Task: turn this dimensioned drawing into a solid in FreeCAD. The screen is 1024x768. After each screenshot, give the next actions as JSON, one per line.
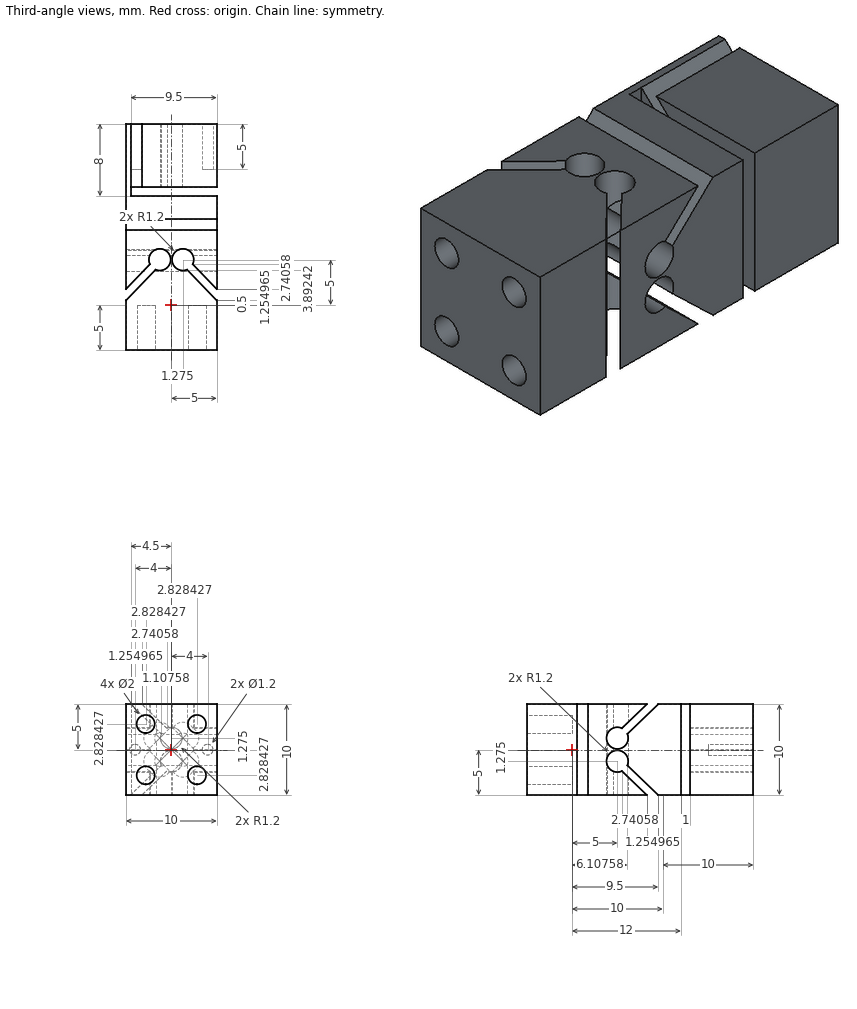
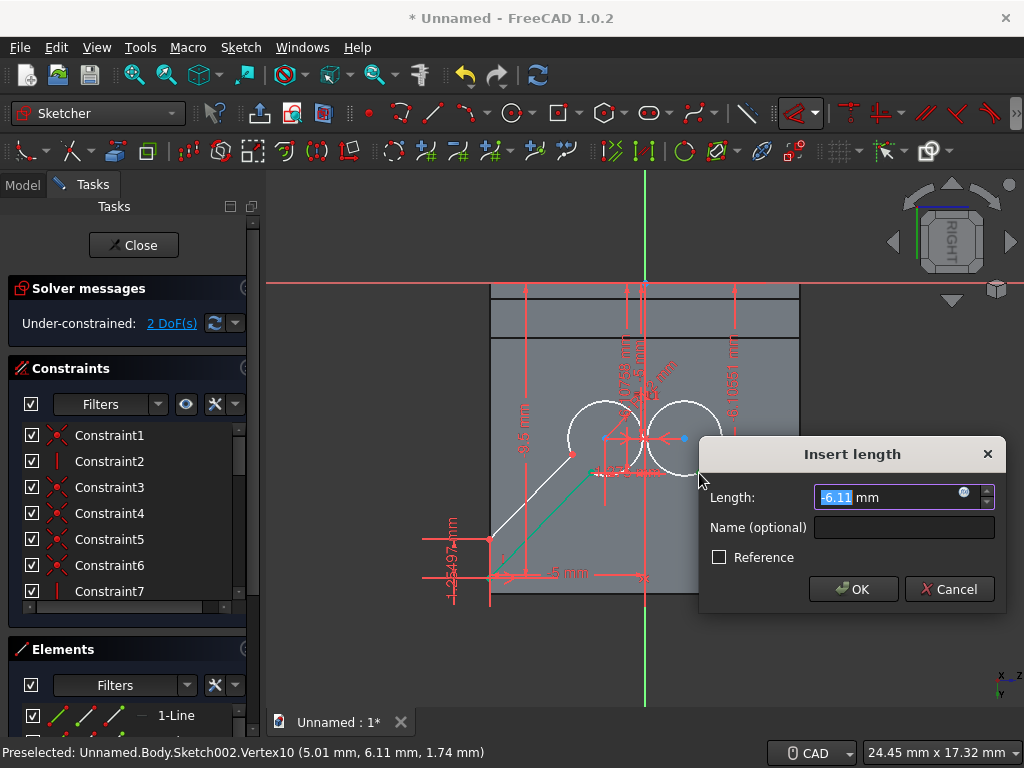
{"action": "type", "text": "-6.10758"}
{"action": "key", "text": "Return"}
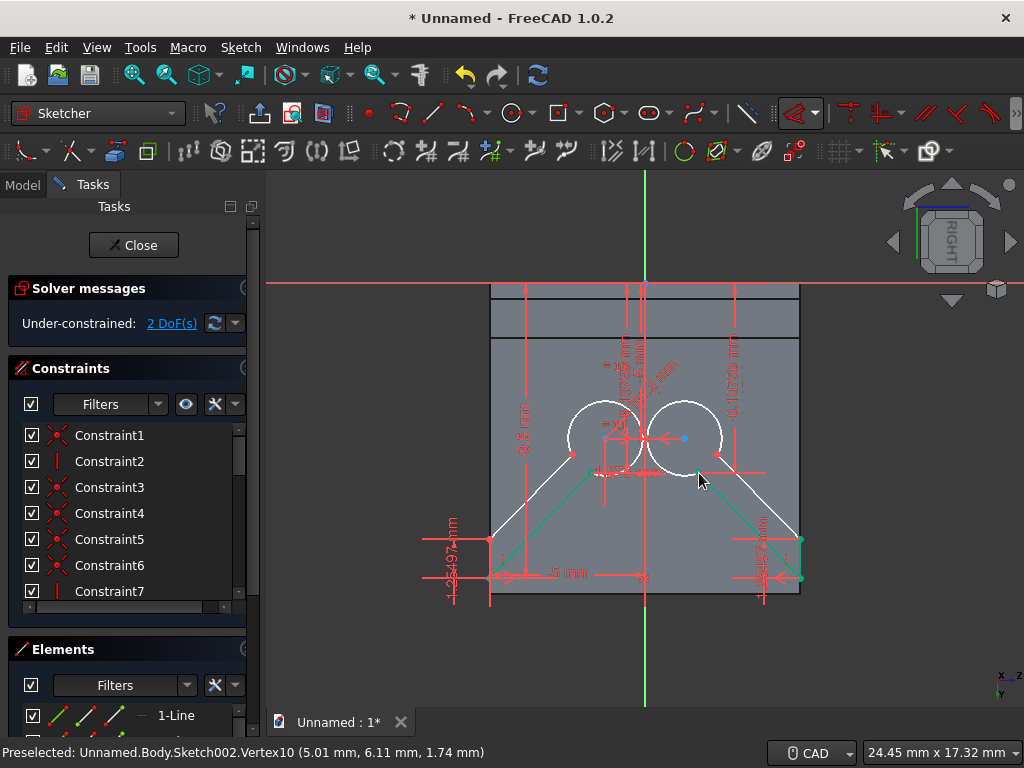
{"action": "left_click", "coordinate": [547, 480]}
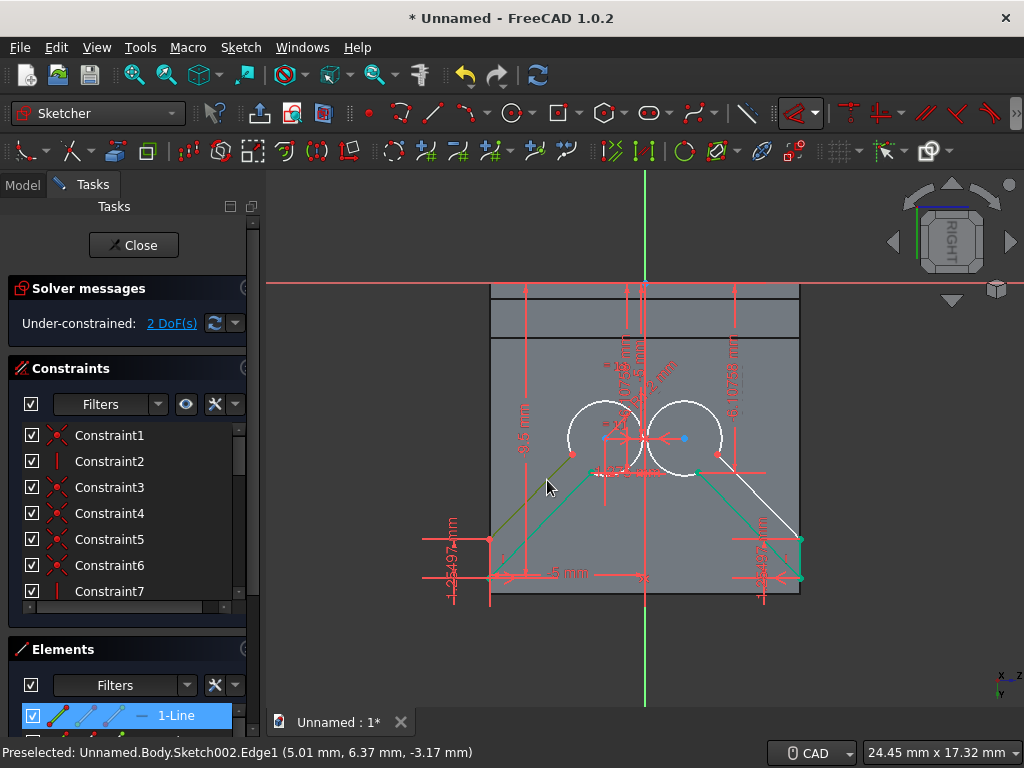
{"action": "left_click", "coordinate": [818, 114]}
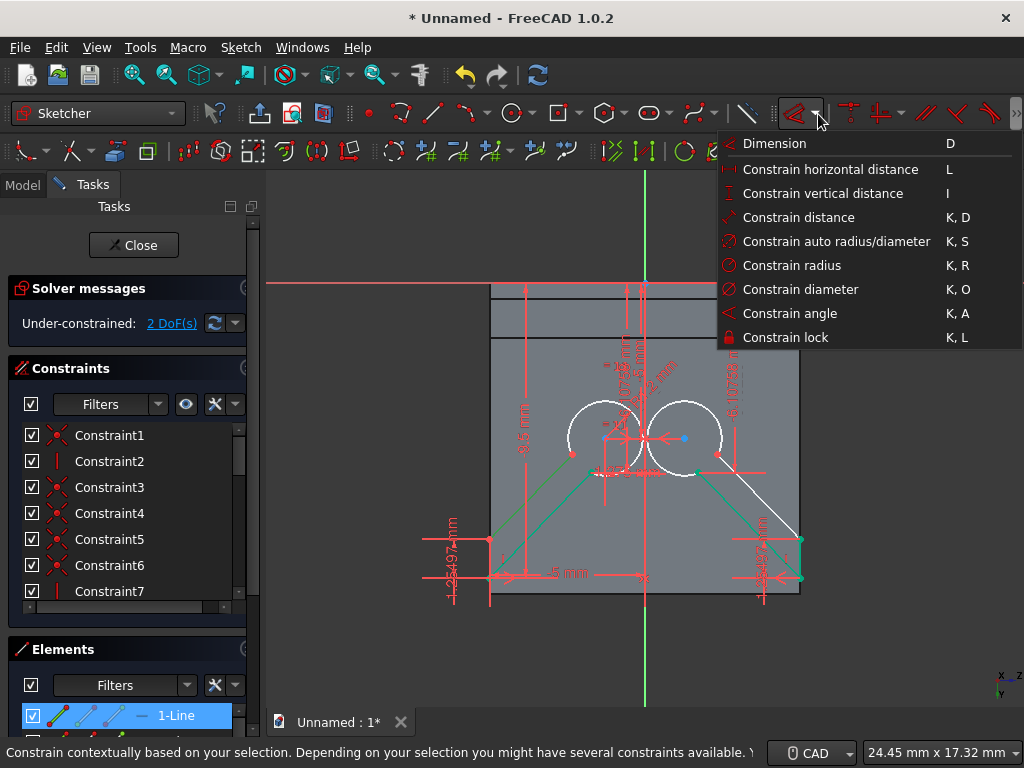
{"action": "left_click", "coordinate": [870, 193]}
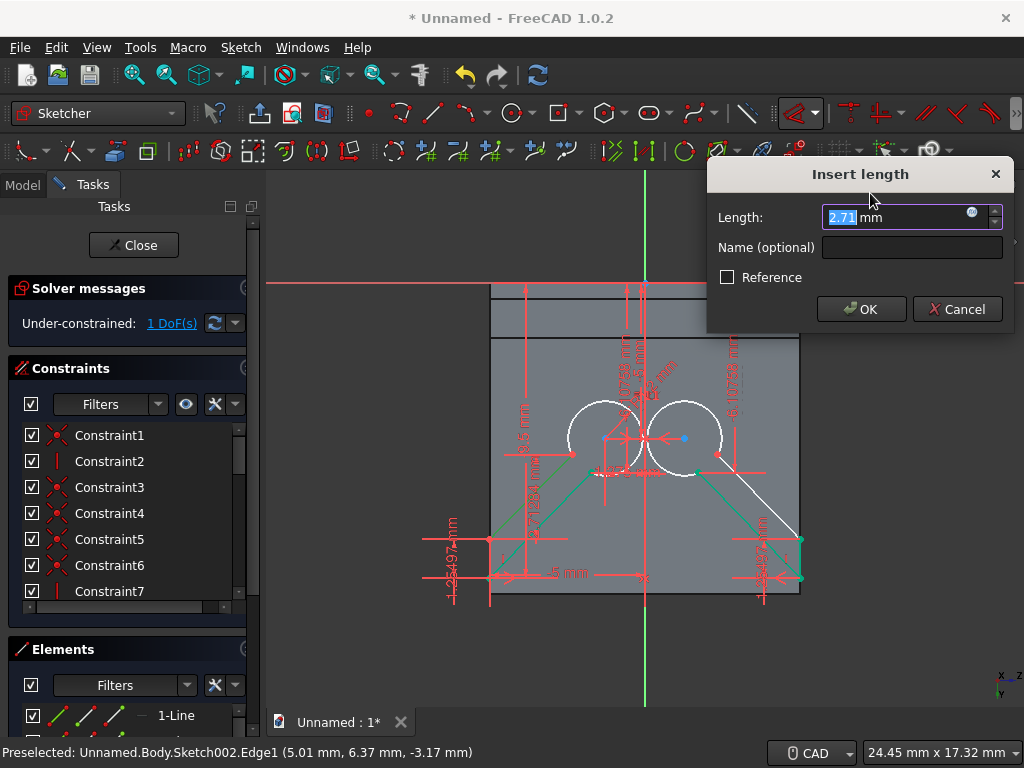
{"action": "type", "text": "2.74058"}
{"action": "key", "text": "Return"}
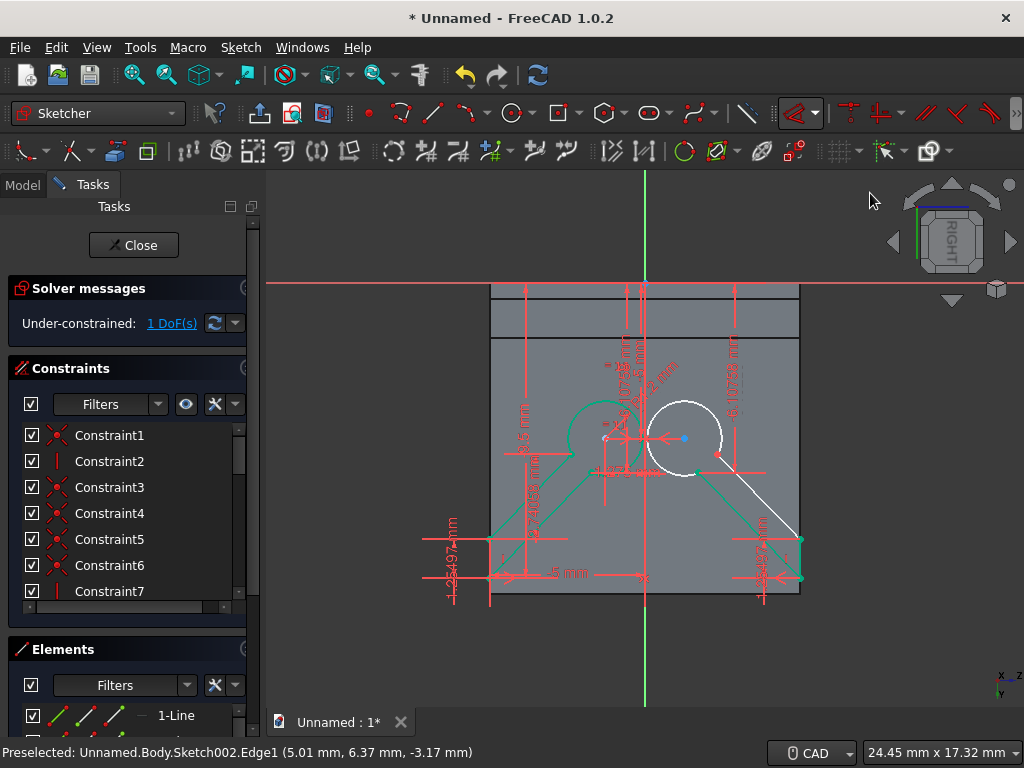
{"action": "left_click", "coordinate": [775, 514]}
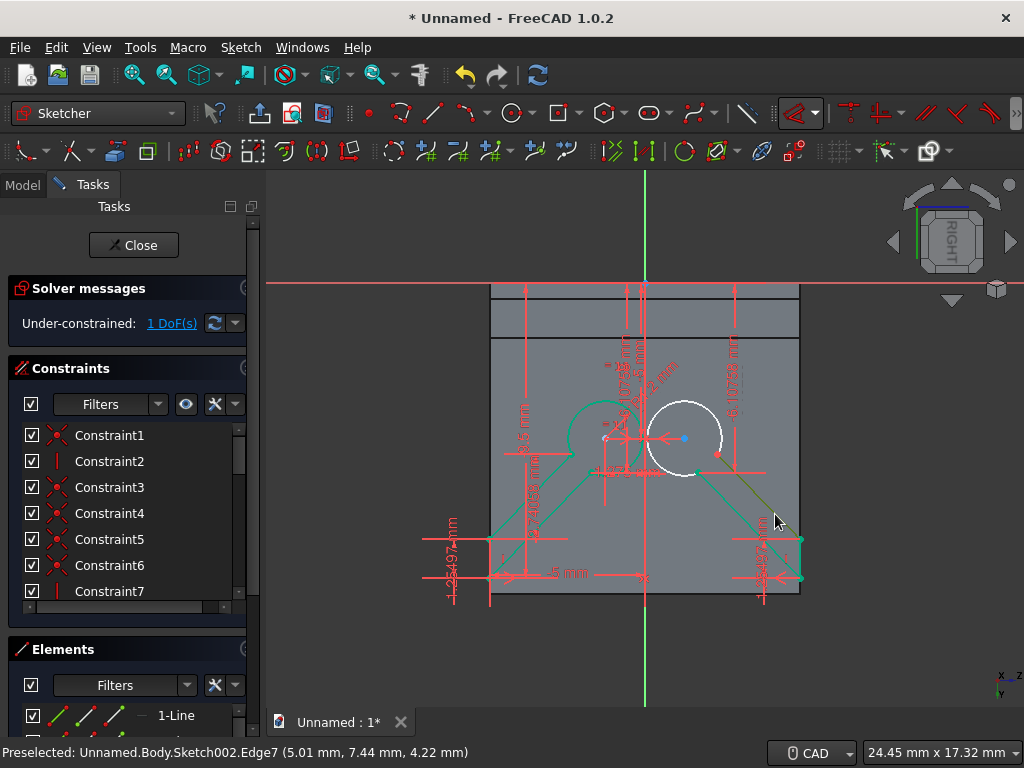
{"action": "left_click", "coordinate": [818, 114]}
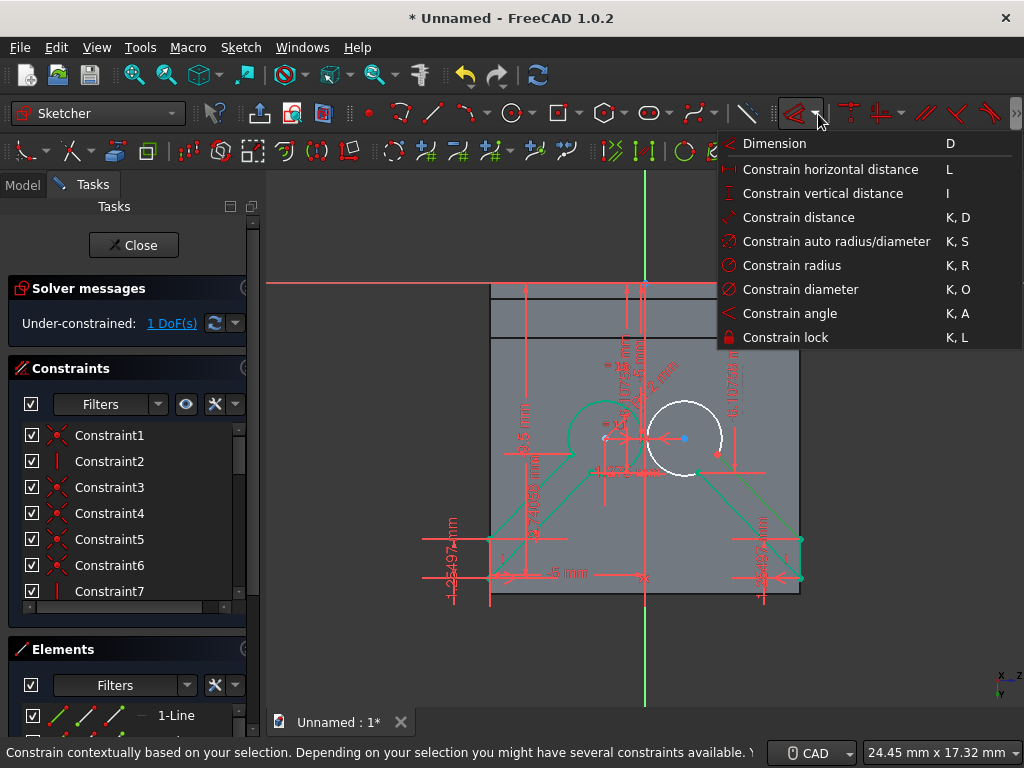
{"action": "left_click", "coordinate": [870, 193]}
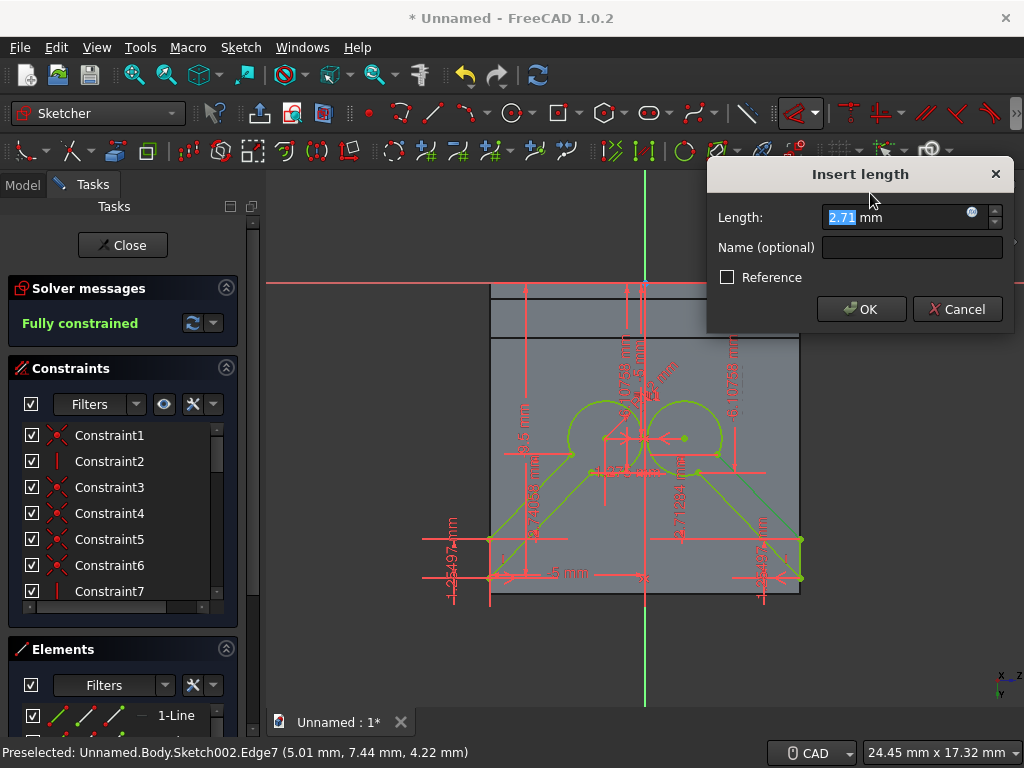
{"action": "type", "text": "2.74058"}
{"action": "key", "text": "Return"}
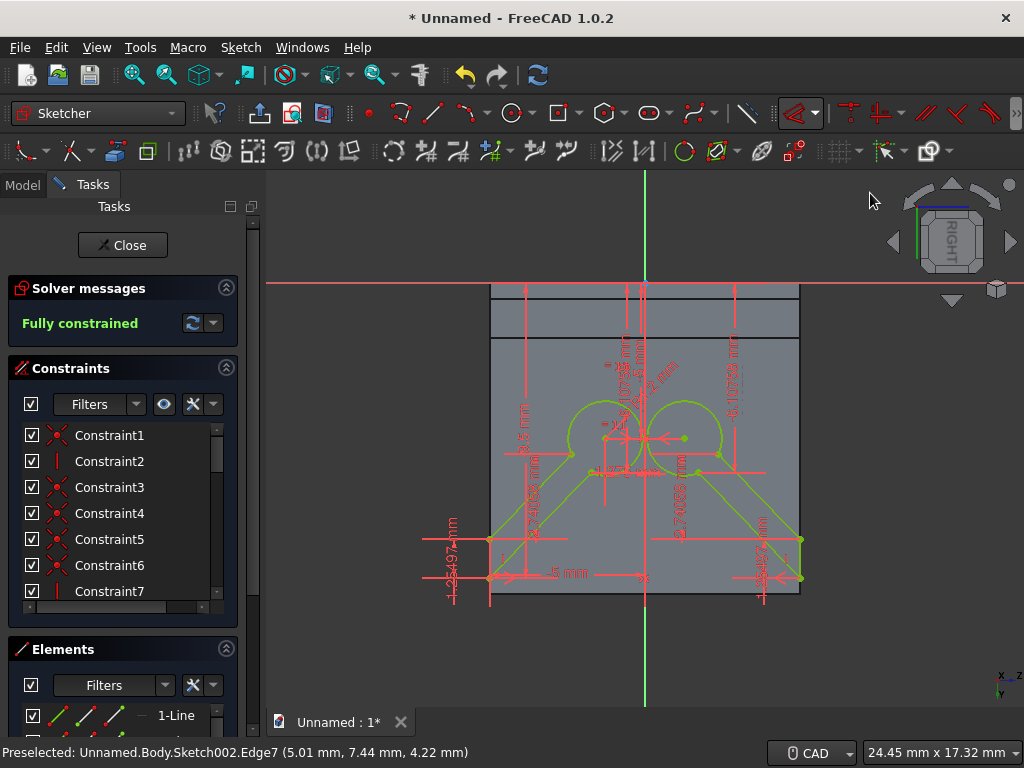
{"action": "left_click", "coordinate": [123, 245]}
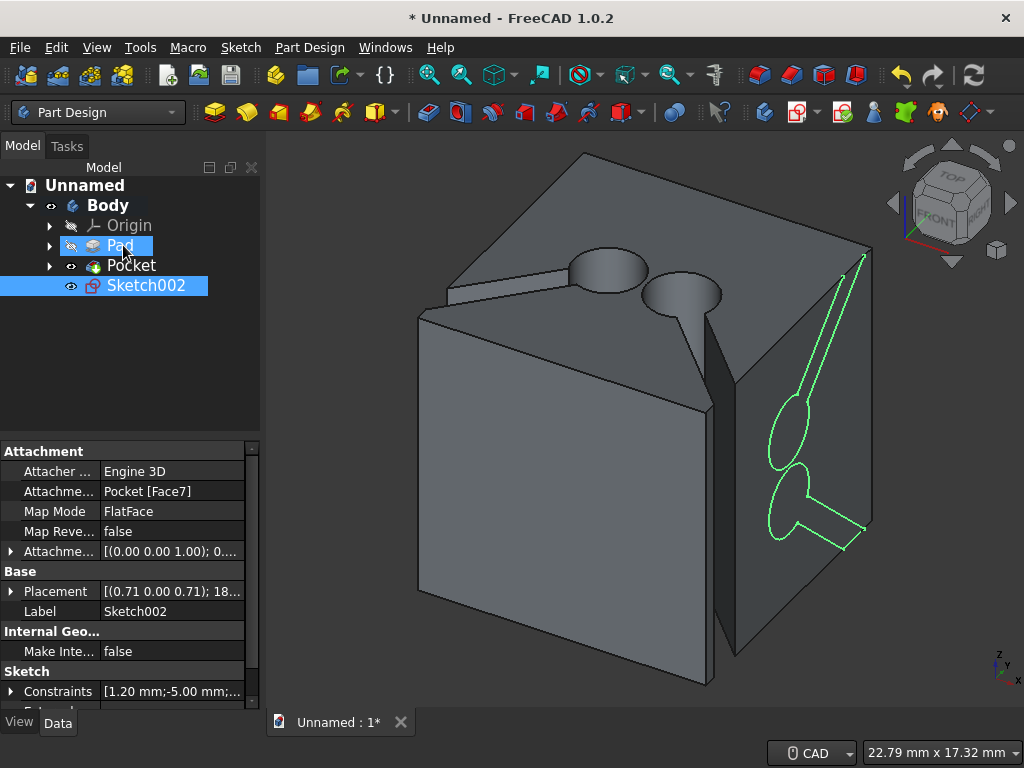
{"action": "left_click", "coordinate": [430, 112]}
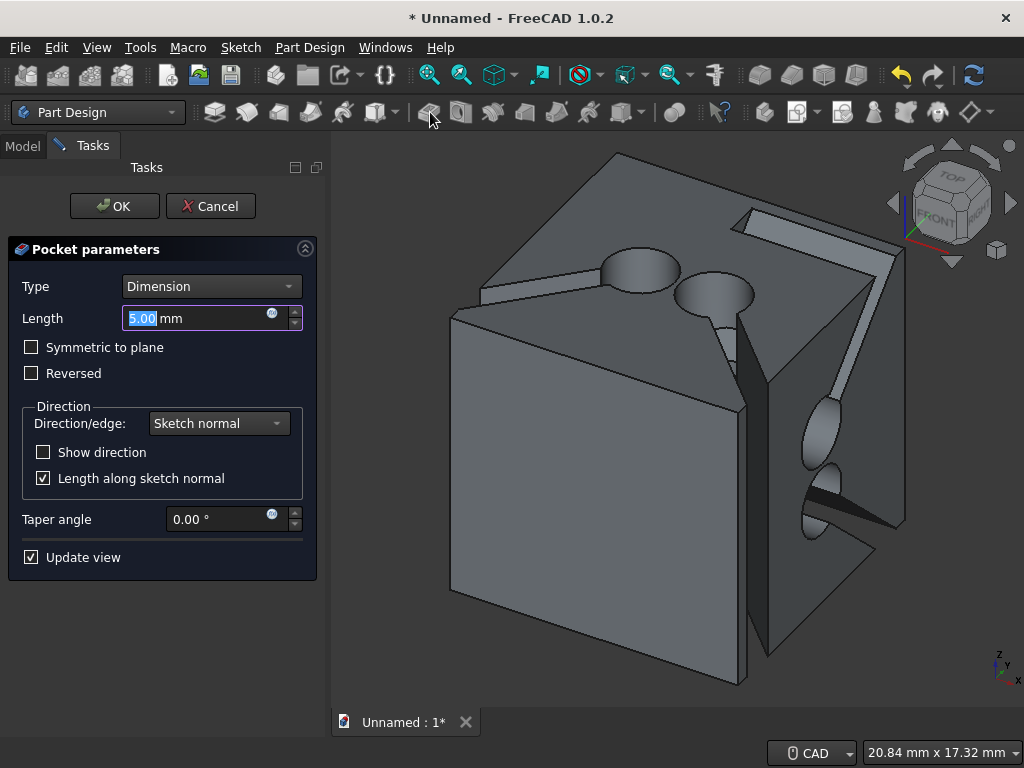
{"action": "left_click", "coordinate": [212, 286]}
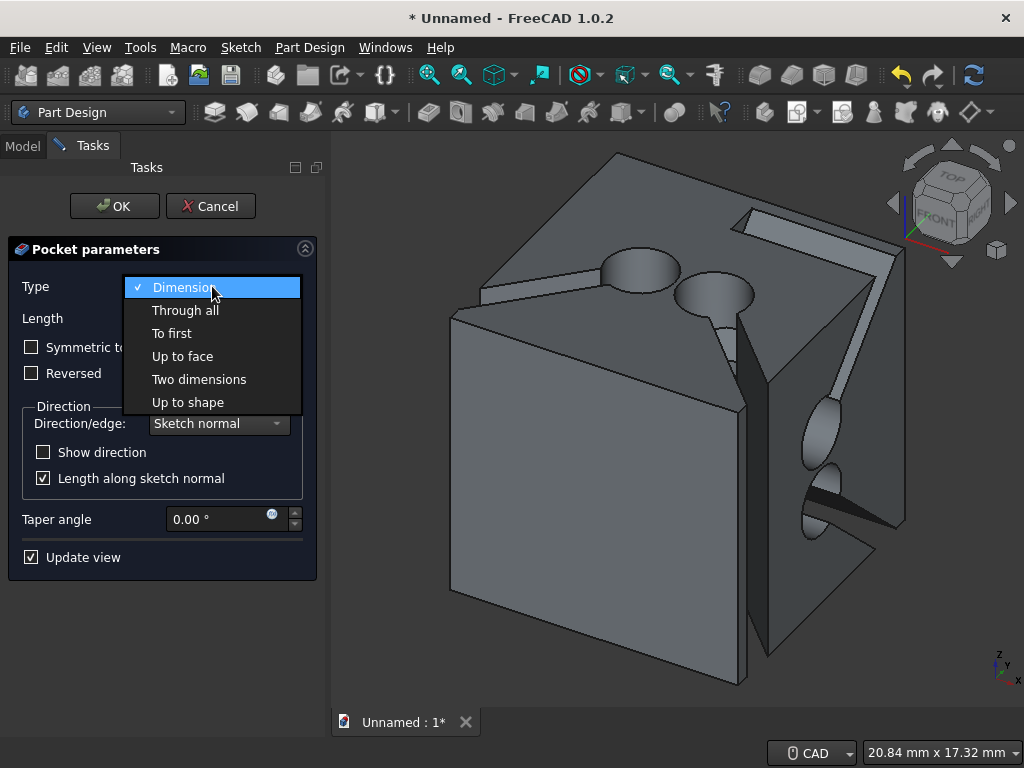
{"action": "left_click", "coordinate": [212, 310]}